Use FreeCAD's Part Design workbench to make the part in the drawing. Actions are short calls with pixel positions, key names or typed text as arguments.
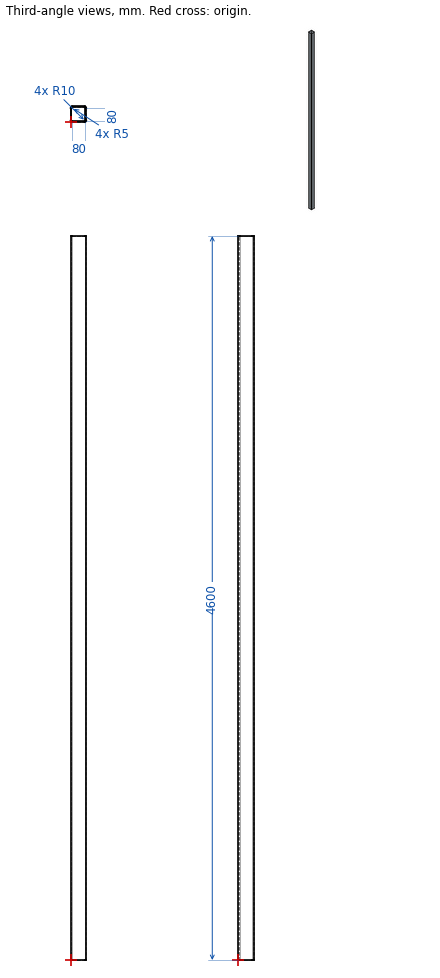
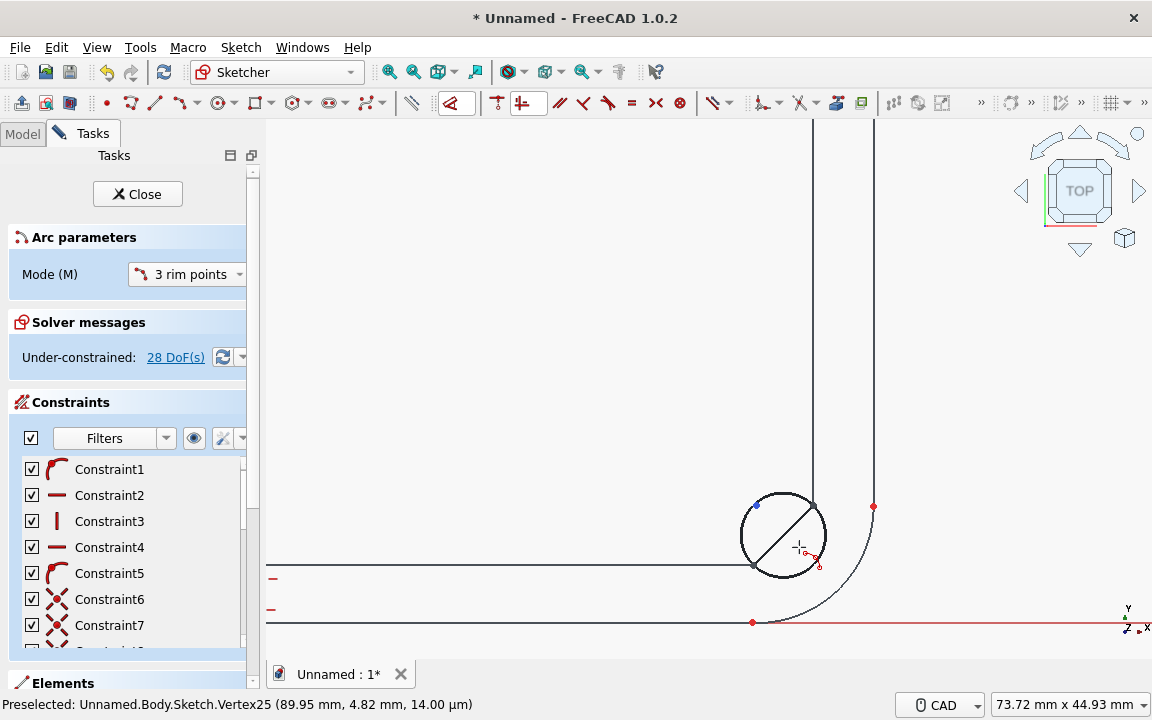
click(797, 545)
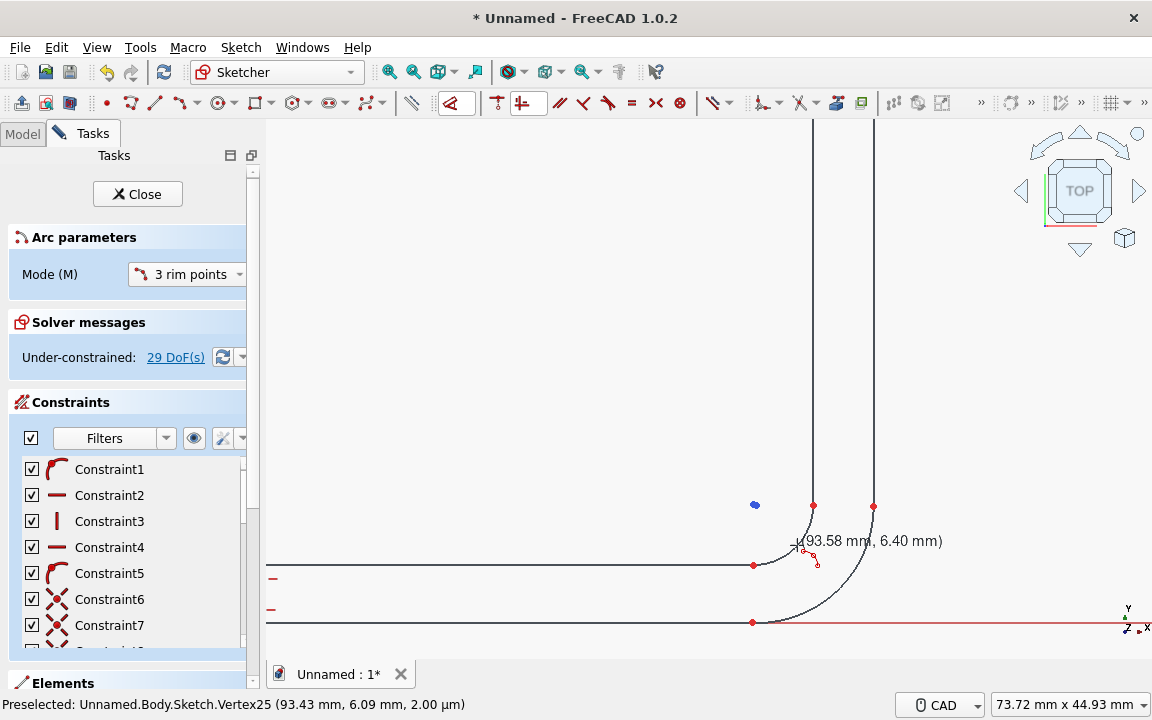
scroll(799, 547, down, 6)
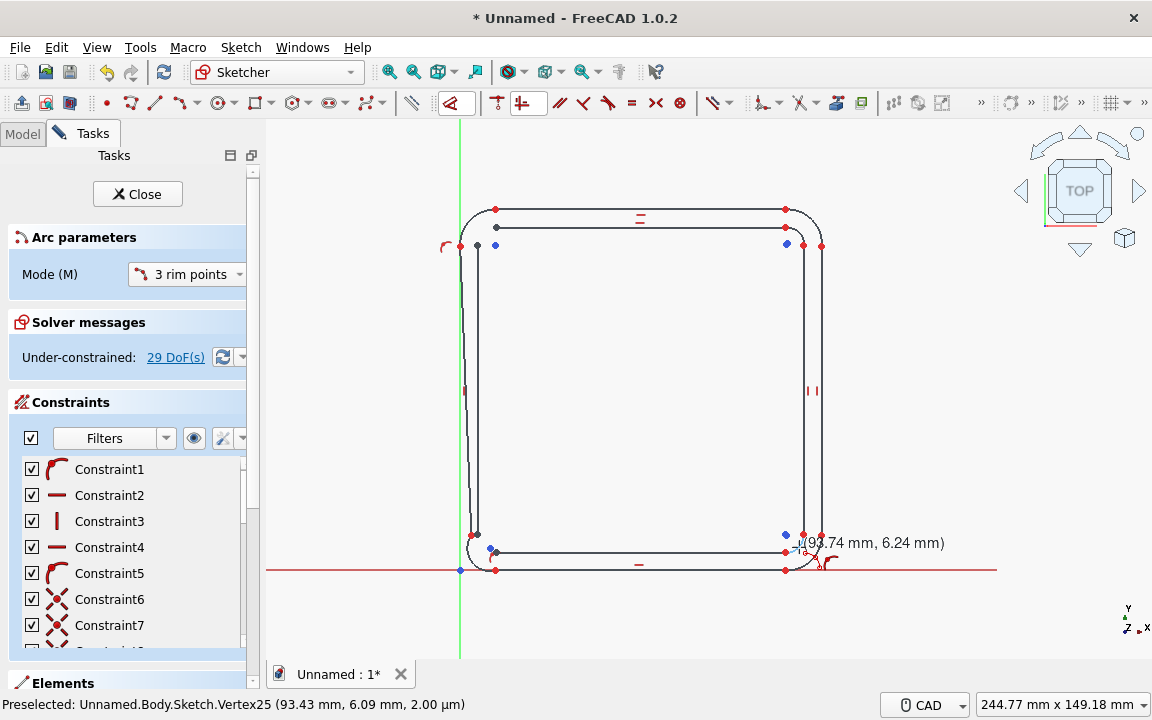
click(497, 553)
click(478, 535)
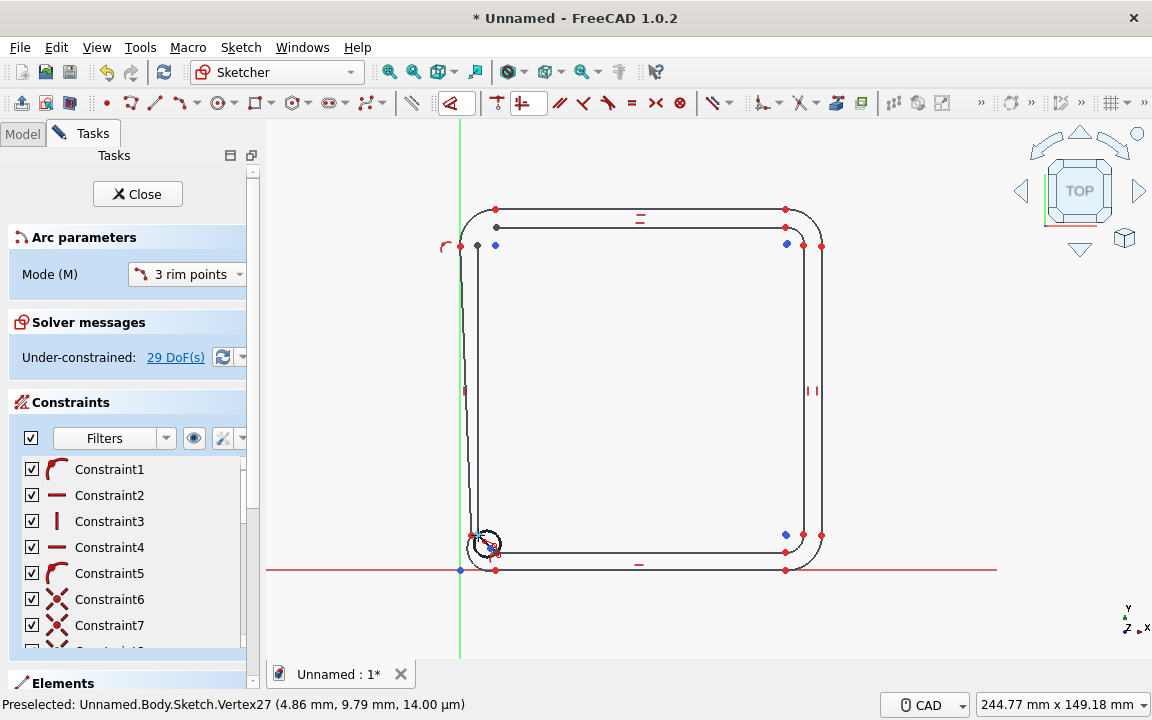
scroll(483, 547, up, 6)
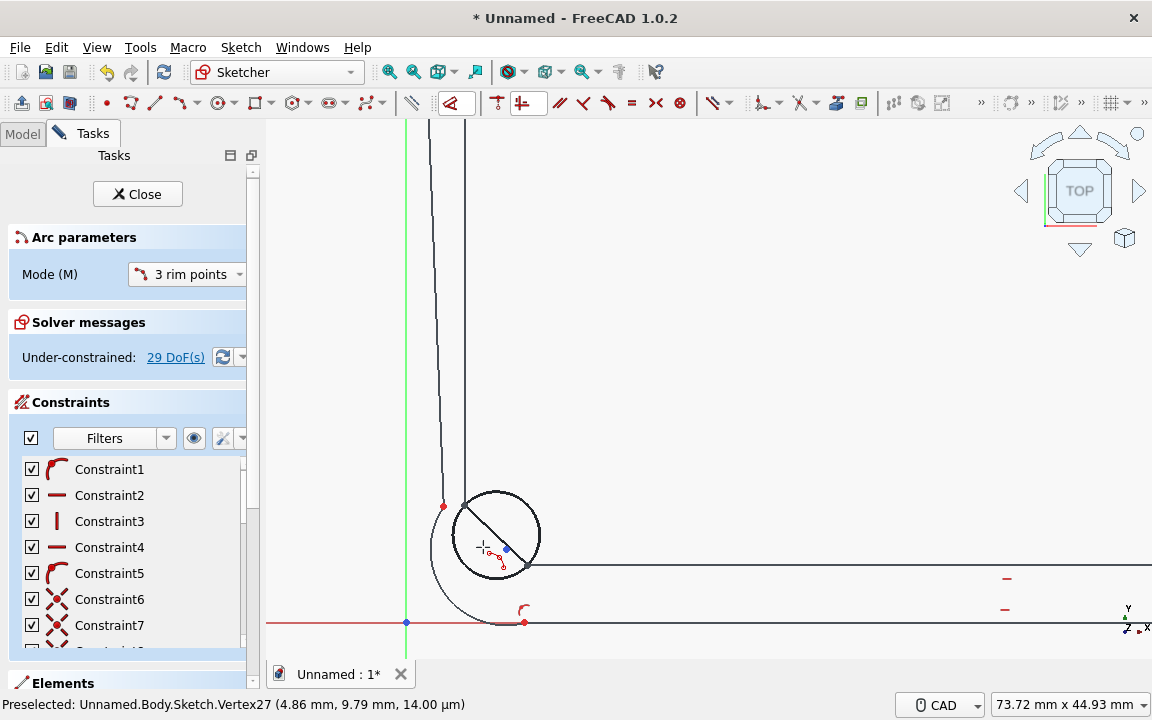
click(484, 545)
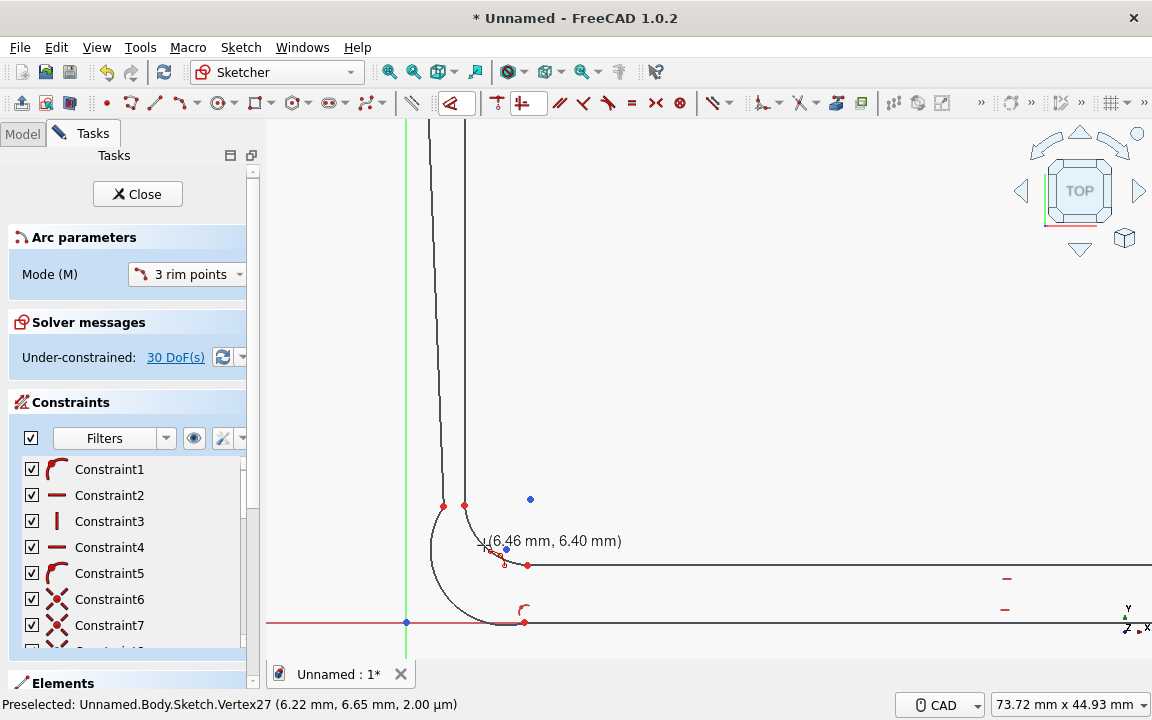
scroll(482, 547, down, 6)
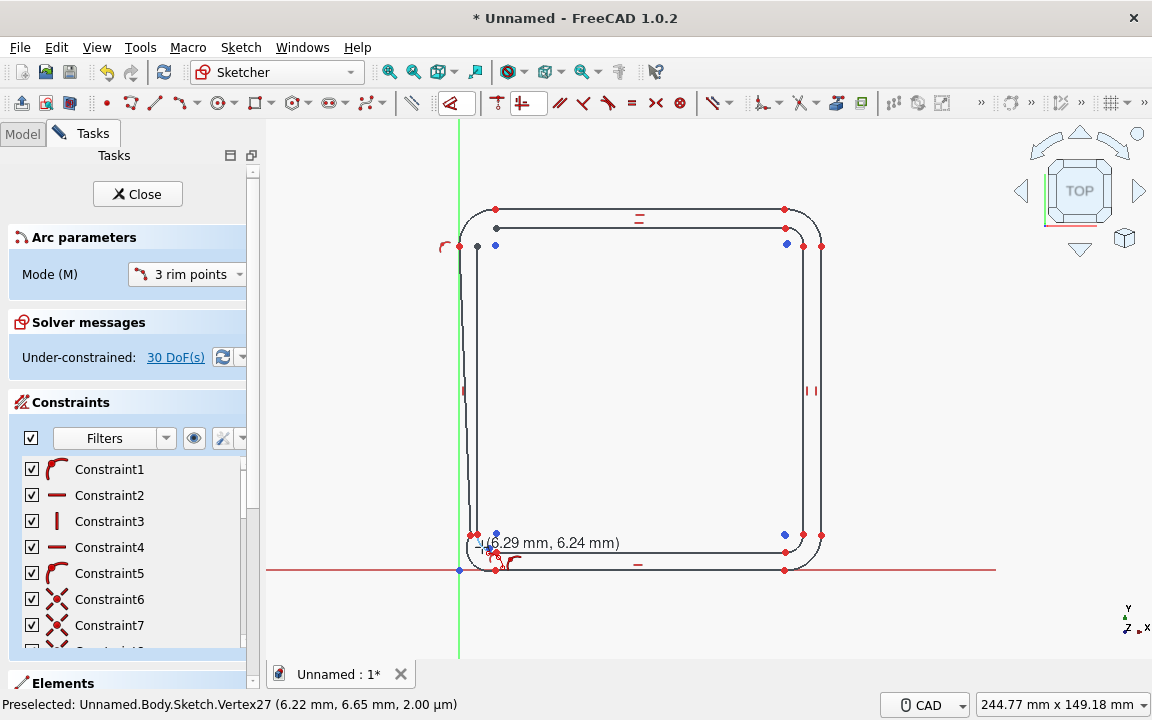
click(477, 246)
click(496, 228)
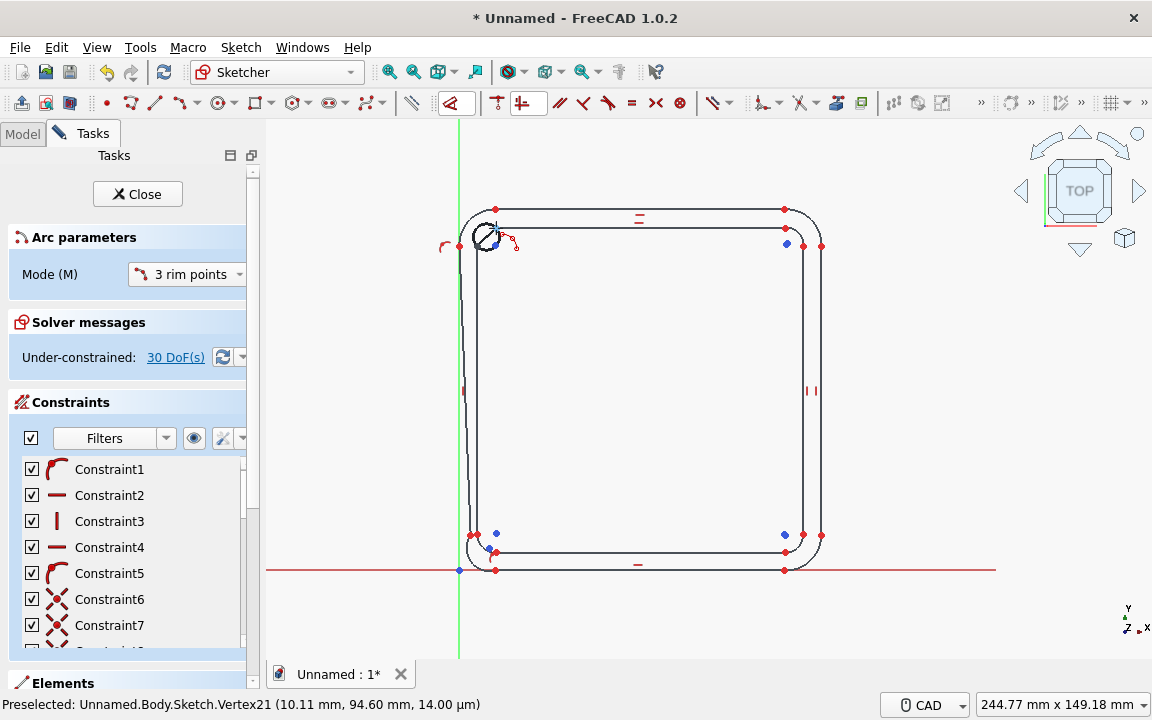
scroll(483, 232, up, 6)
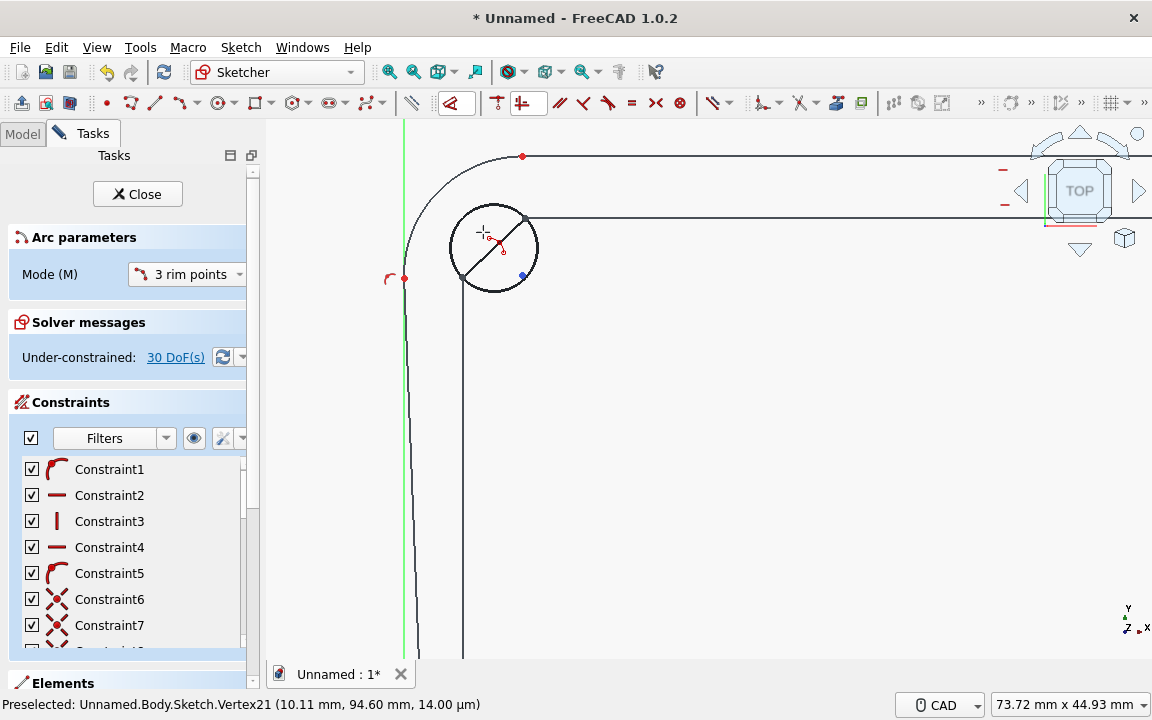
click(482, 231)
key(Escape)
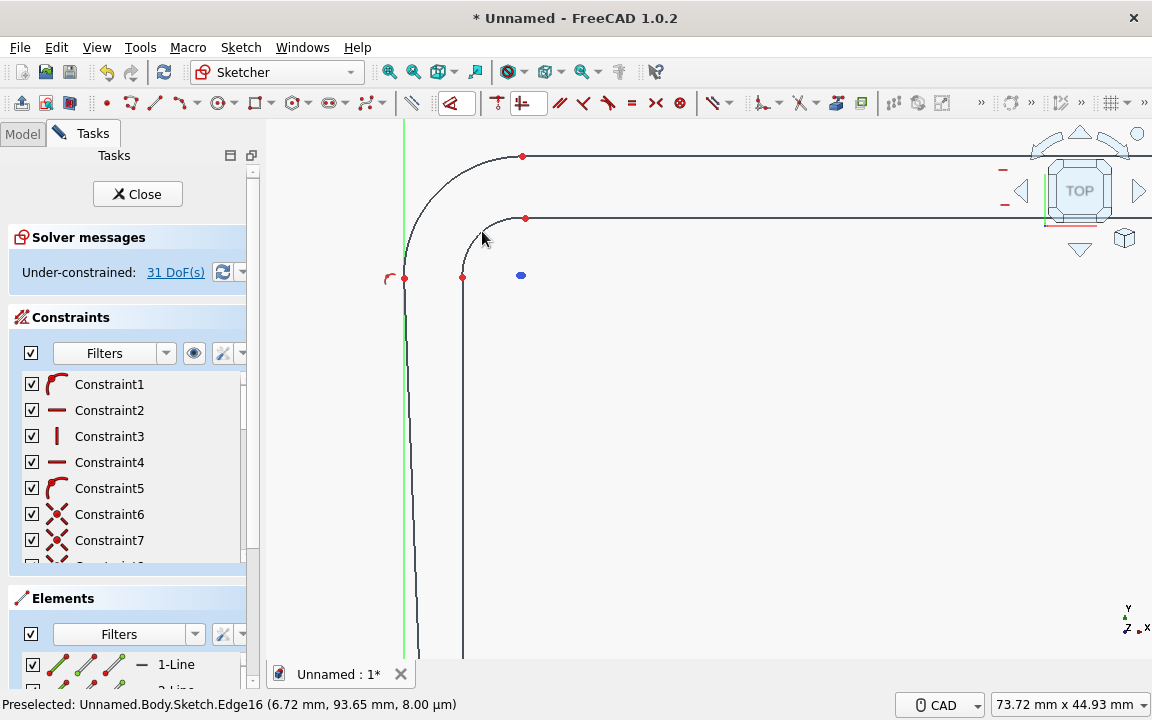
scroll(483, 232, down, 6)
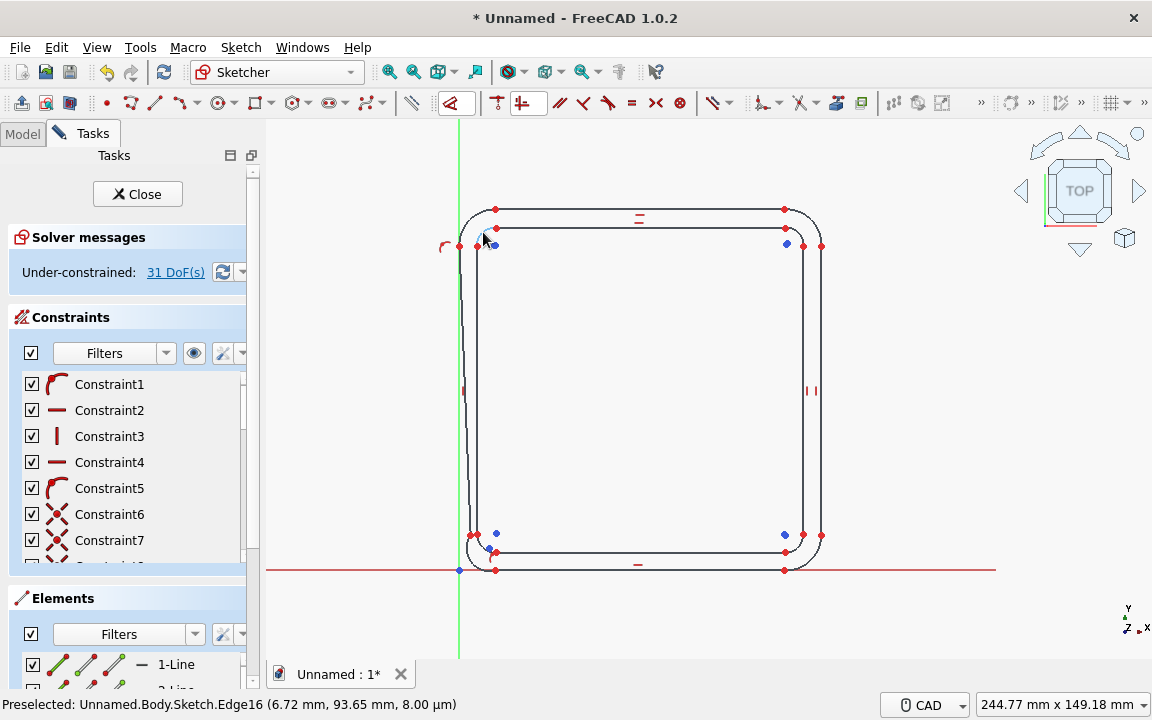
click(582, 570)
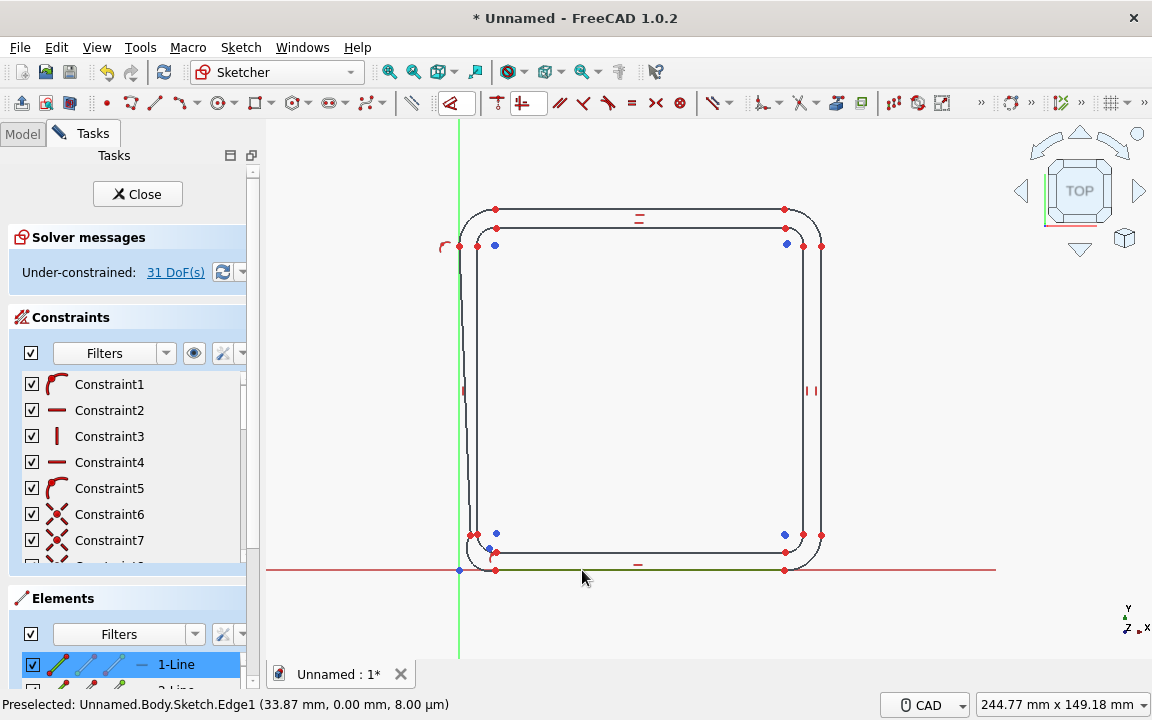
click(801, 567)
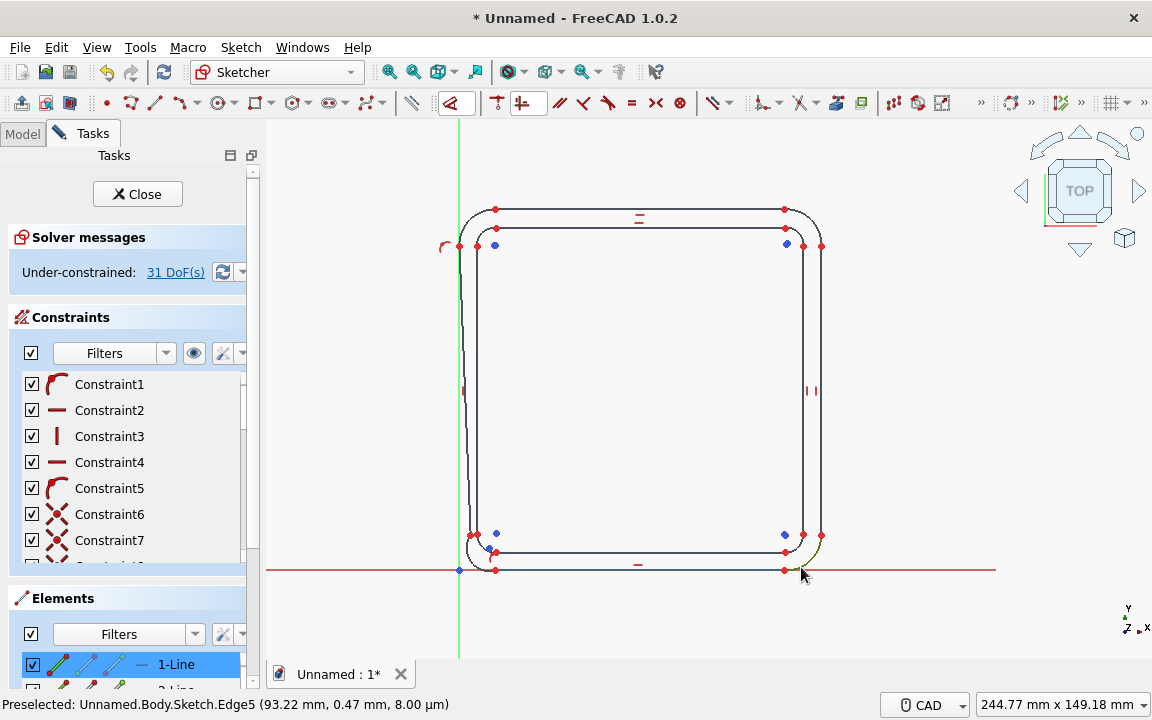
key(t)